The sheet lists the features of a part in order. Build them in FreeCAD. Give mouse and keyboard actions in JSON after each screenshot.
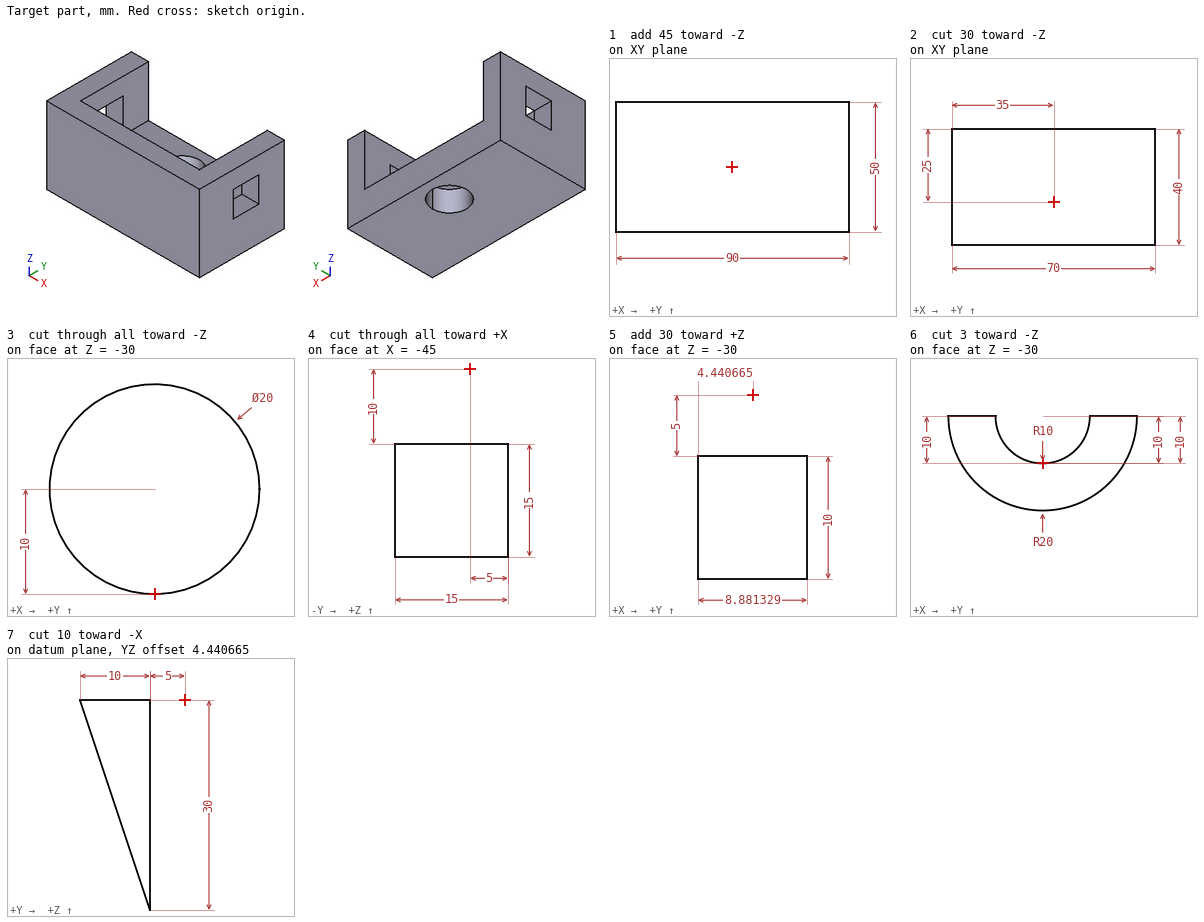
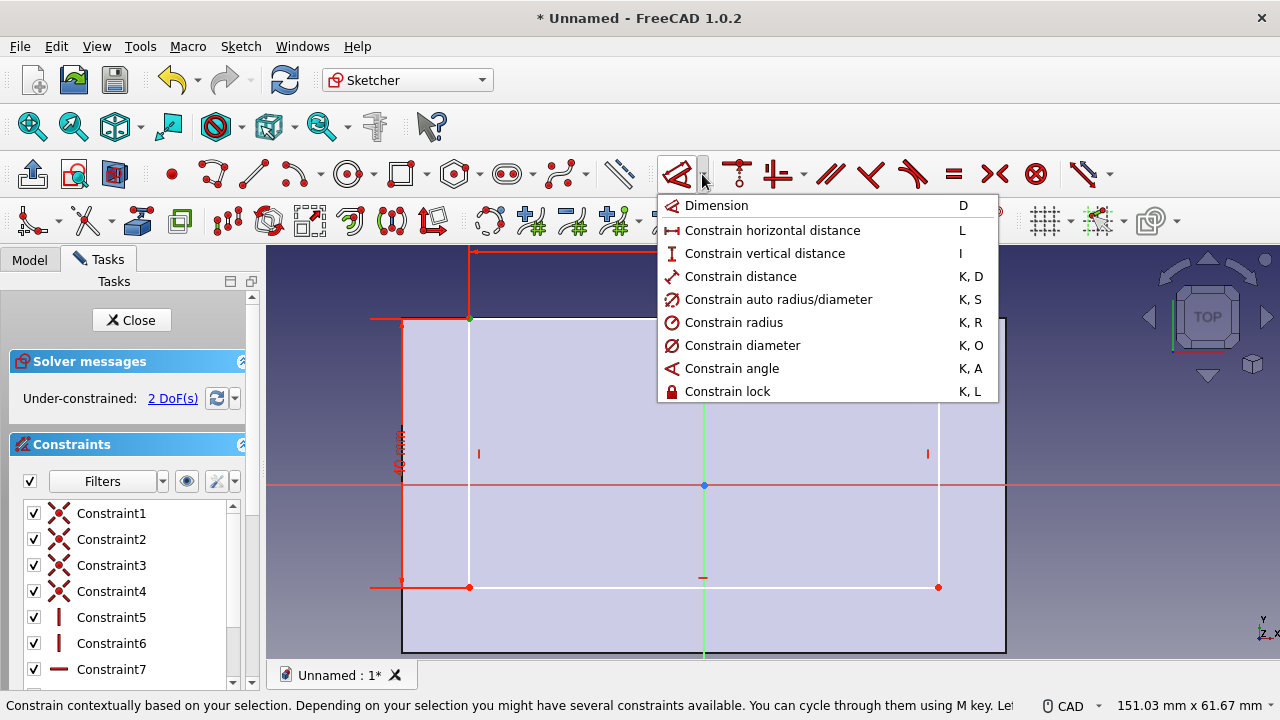
{"action": "left_click", "coordinate": [828, 230]}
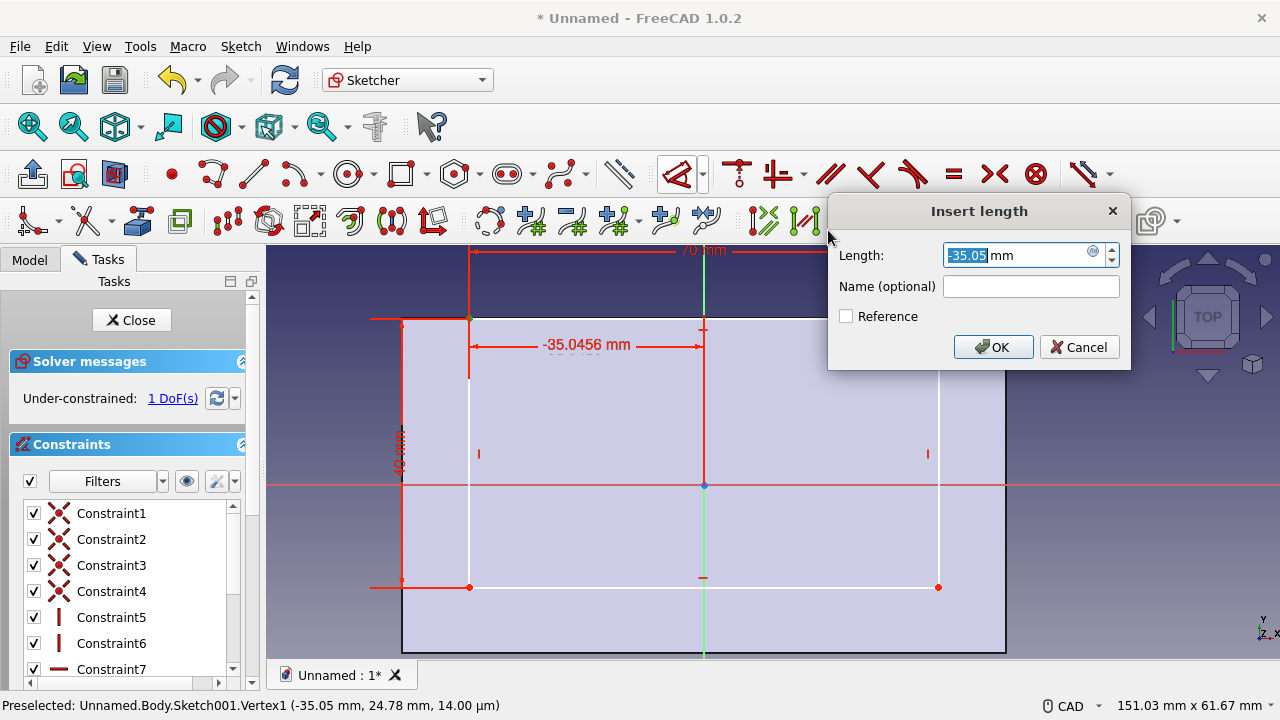
{"action": "type", "text": "-35"}
{"action": "key", "text": "Return"}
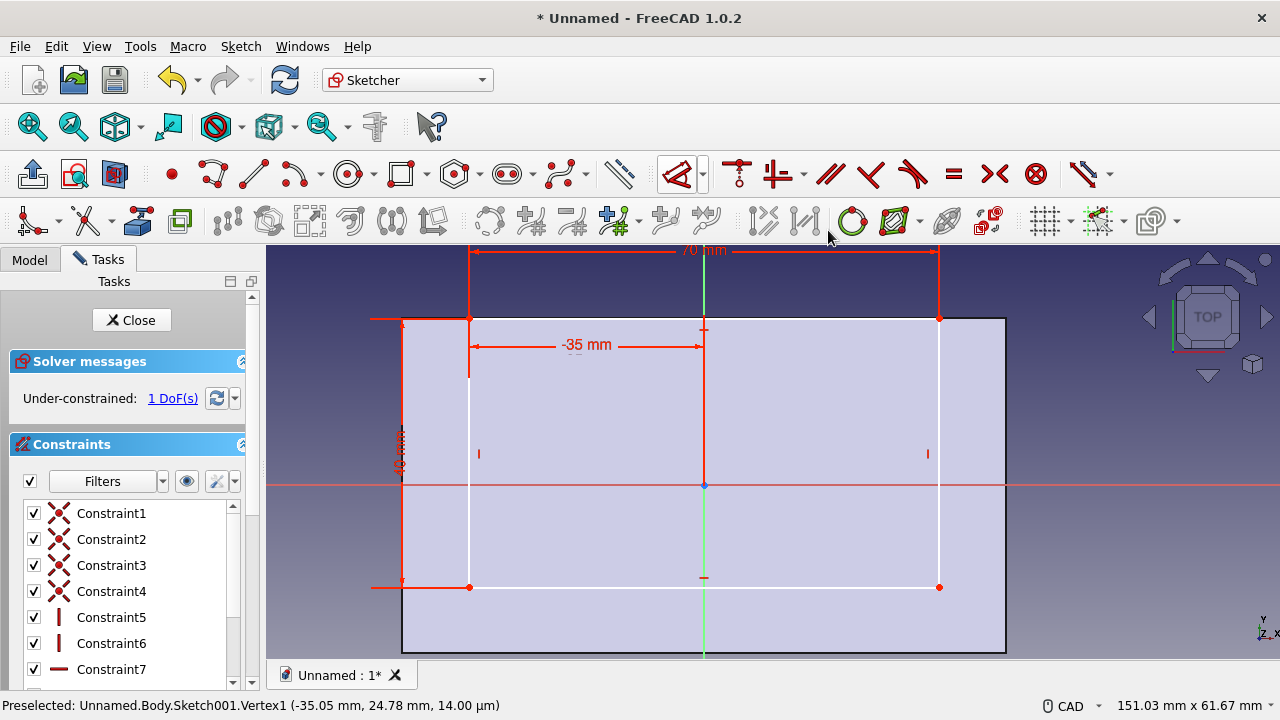
{"action": "left_click", "coordinate": [469, 319]}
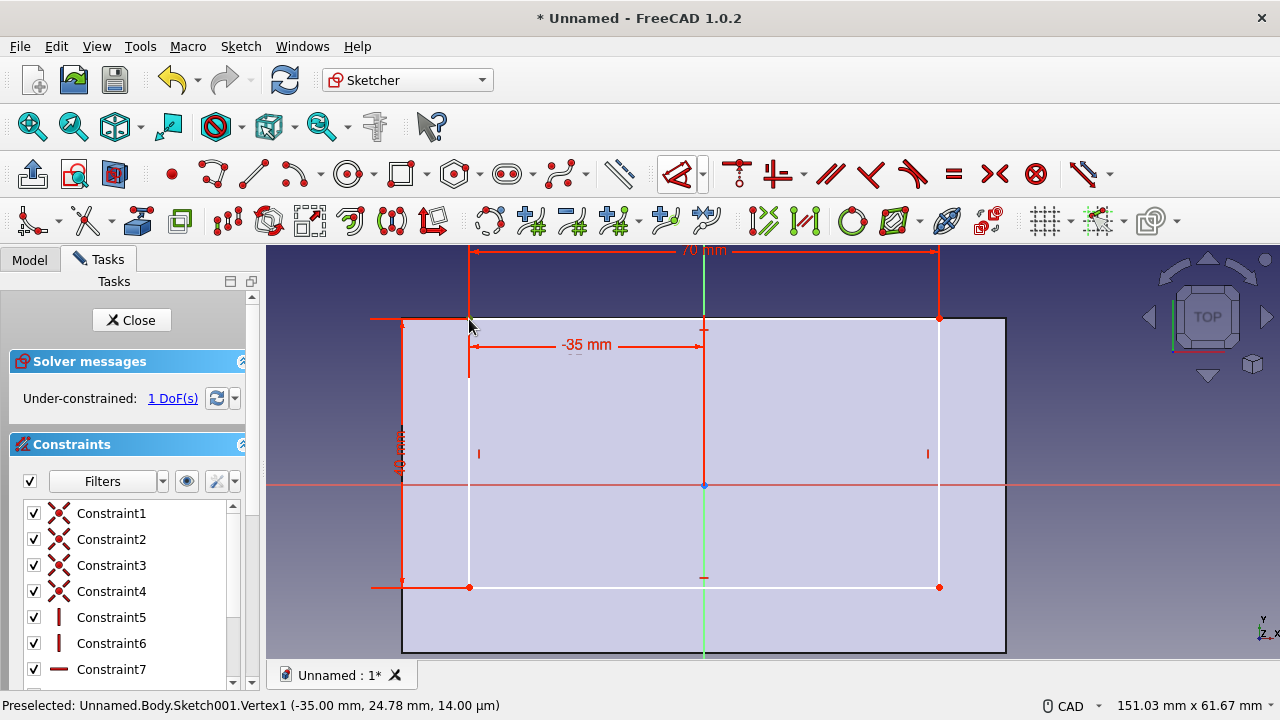
{"action": "key", "text": "i"}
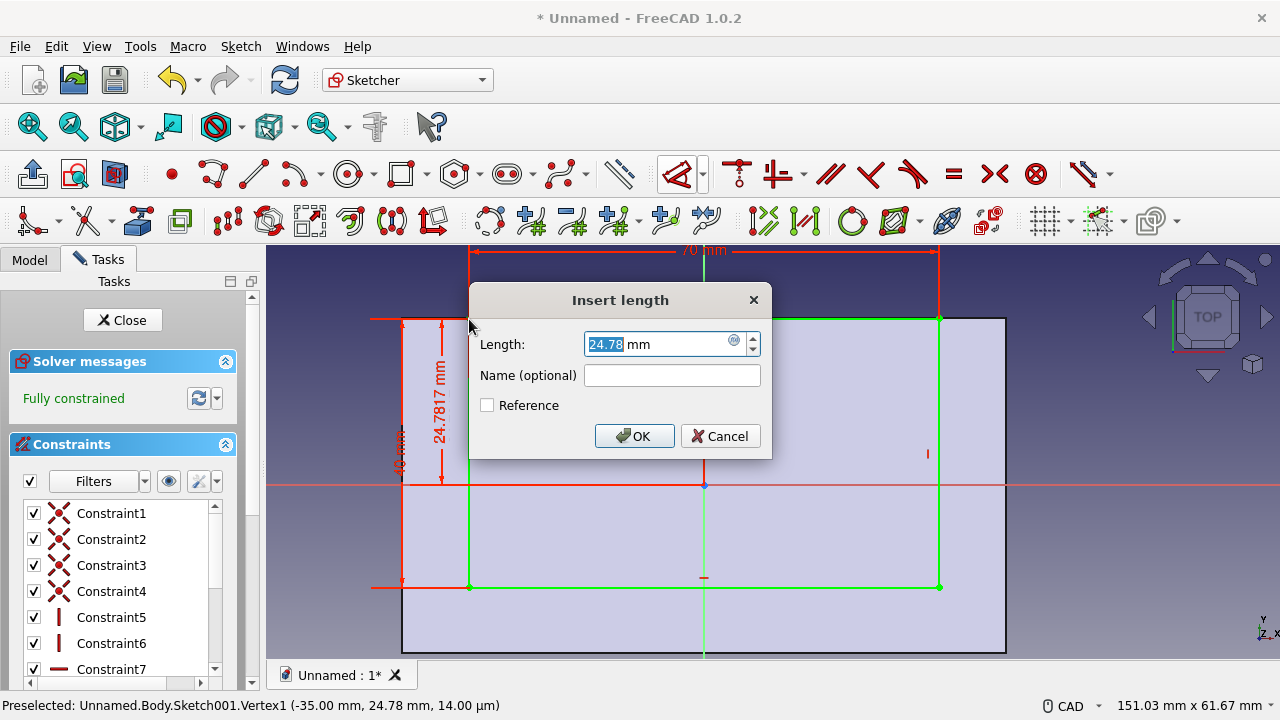
{"action": "type", "text": "25"}
{"action": "key", "text": "Return"}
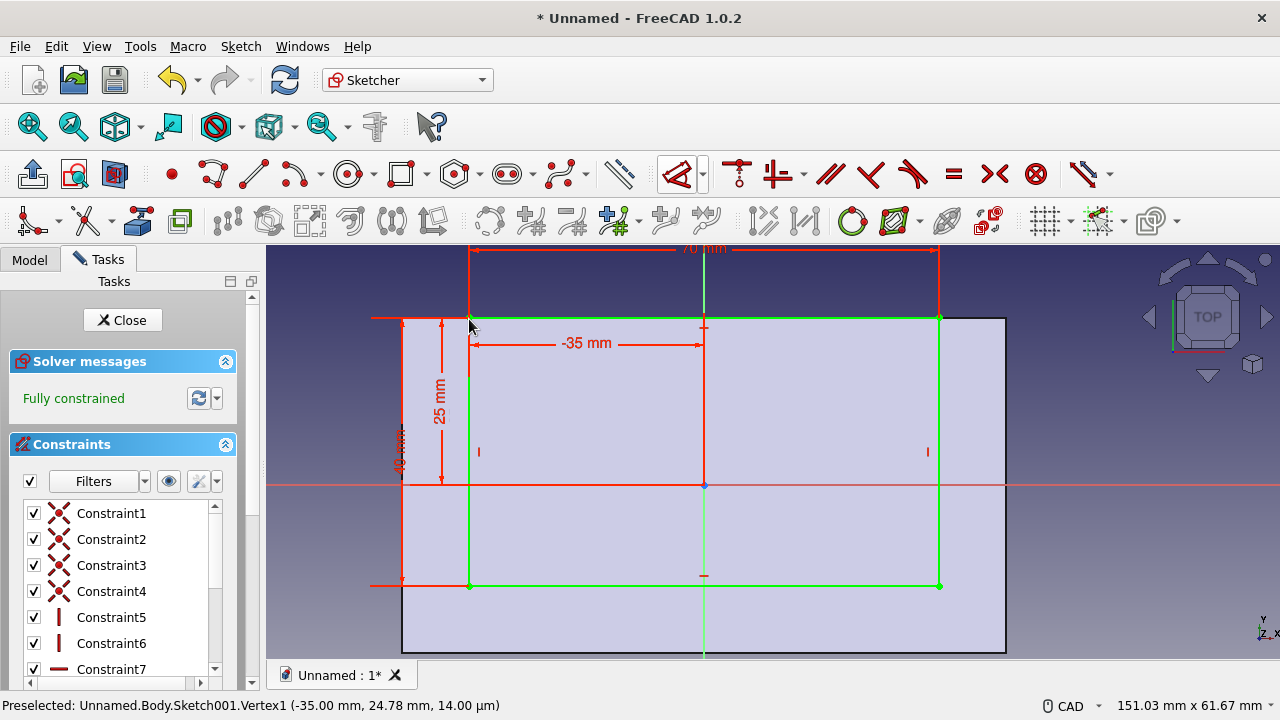
{"action": "left_click", "coordinate": [123, 320]}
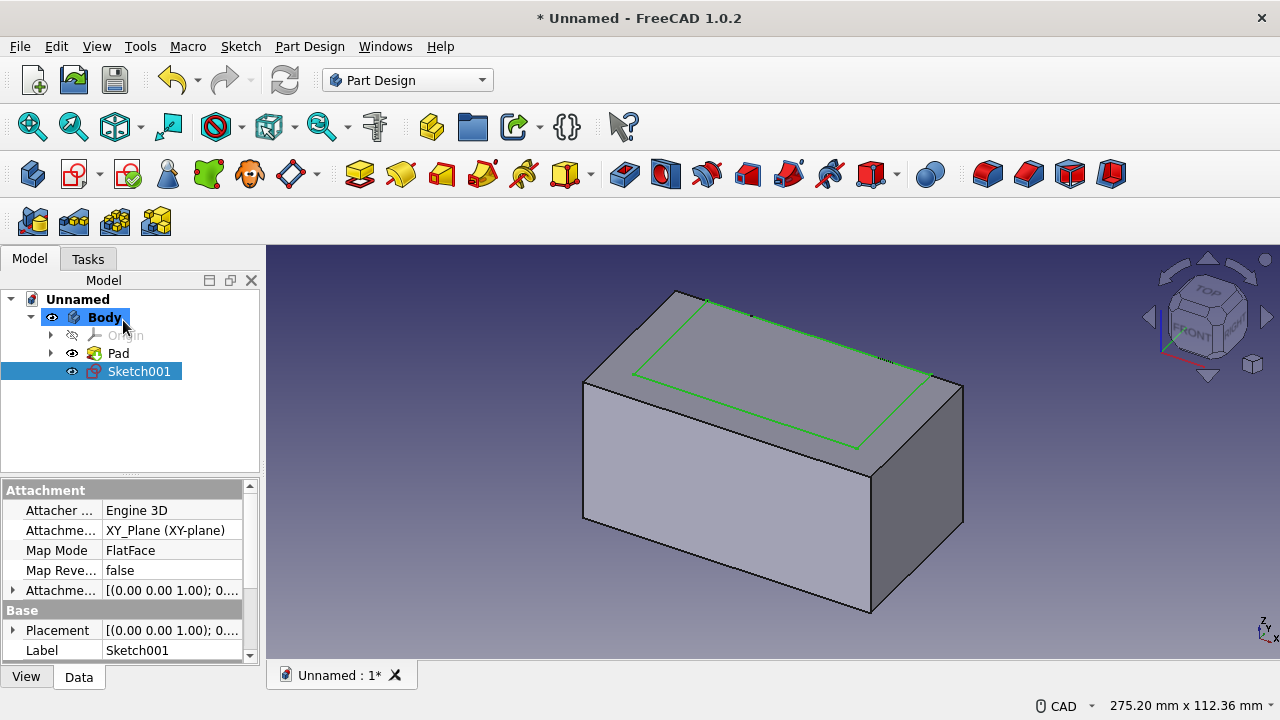
{"action": "left_click", "coordinate": [625, 174]}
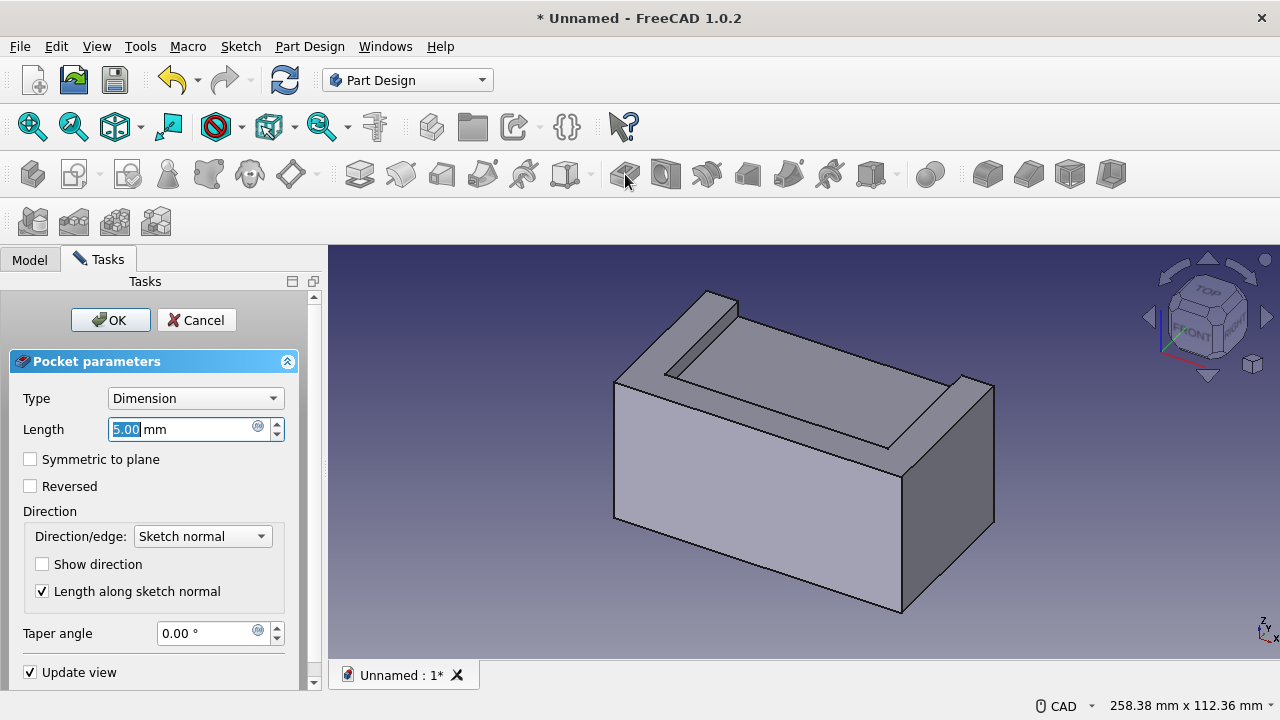
{"action": "type", "text": "30"}
{"action": "key", "text": "Tab"}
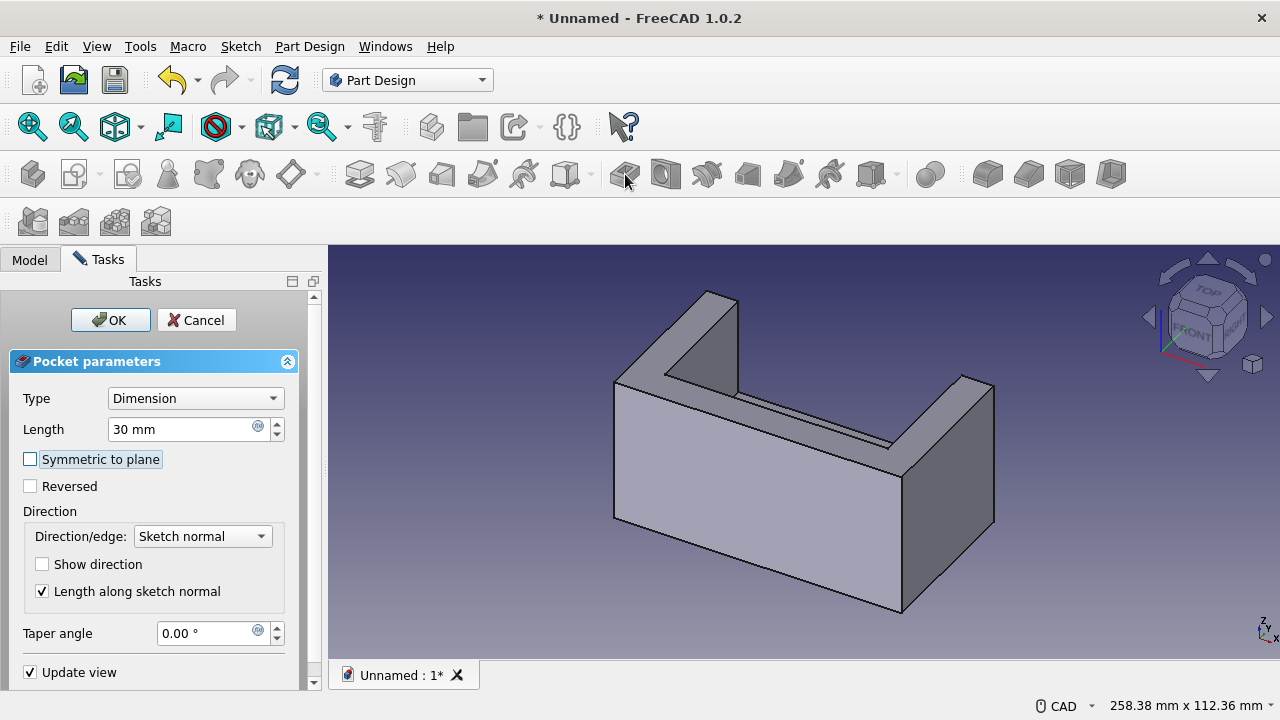
{"action": "left_click", "coordinate": [111, 320]}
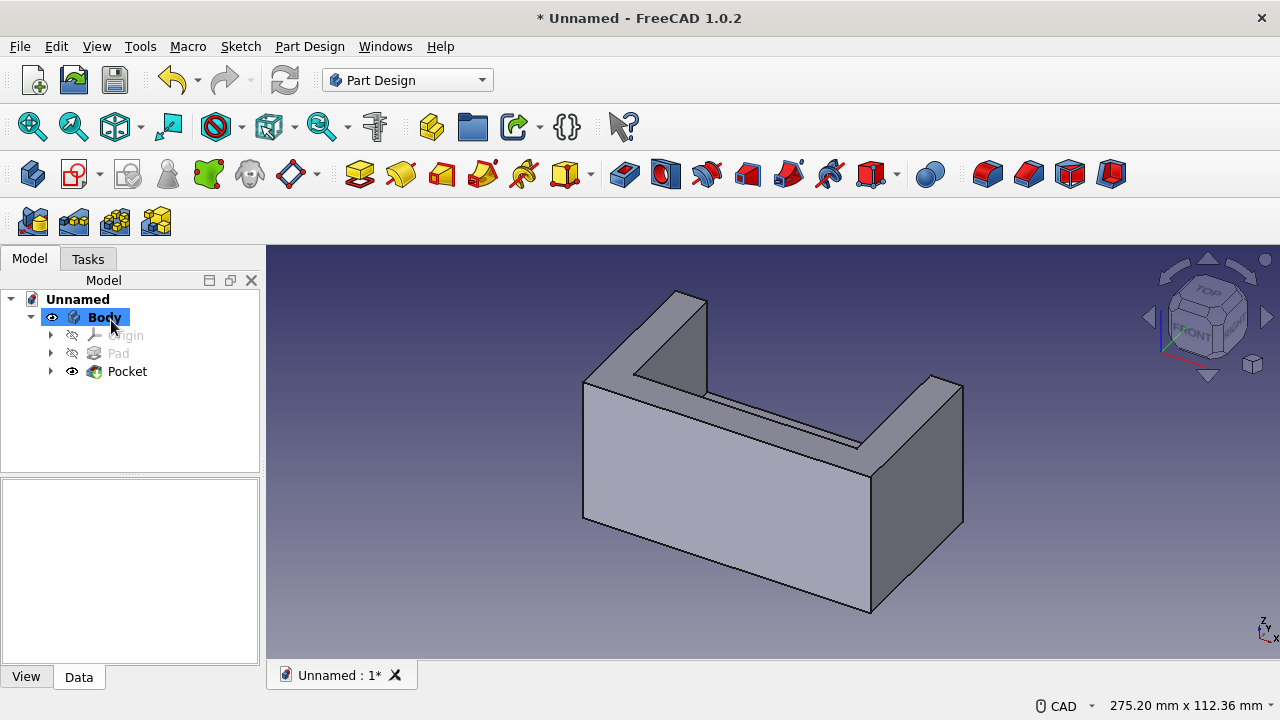
{"action": "key", "text": "0"}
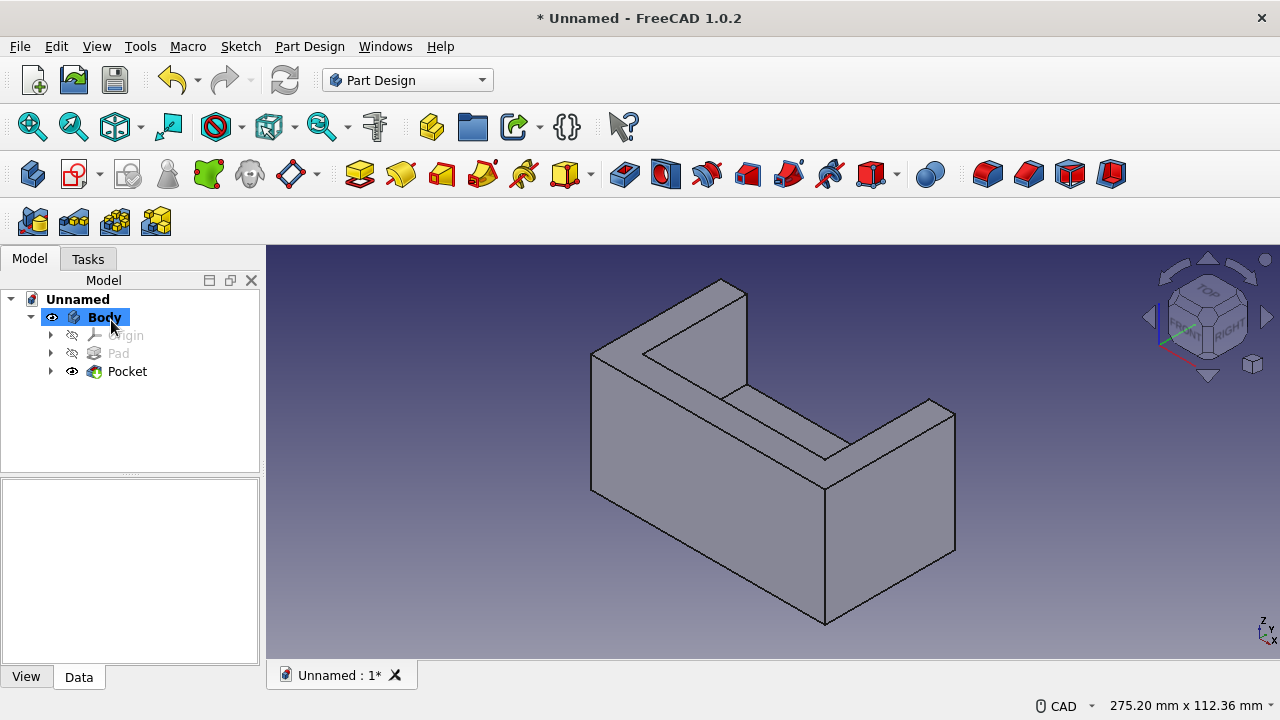
{"action": "key", "text": "2"}